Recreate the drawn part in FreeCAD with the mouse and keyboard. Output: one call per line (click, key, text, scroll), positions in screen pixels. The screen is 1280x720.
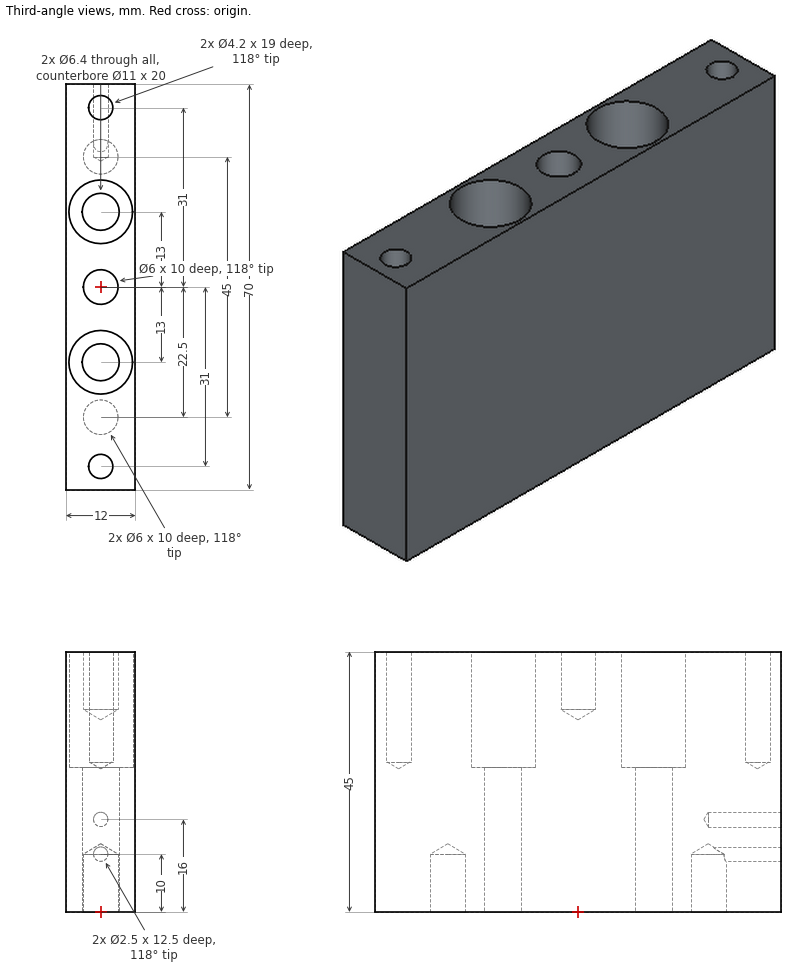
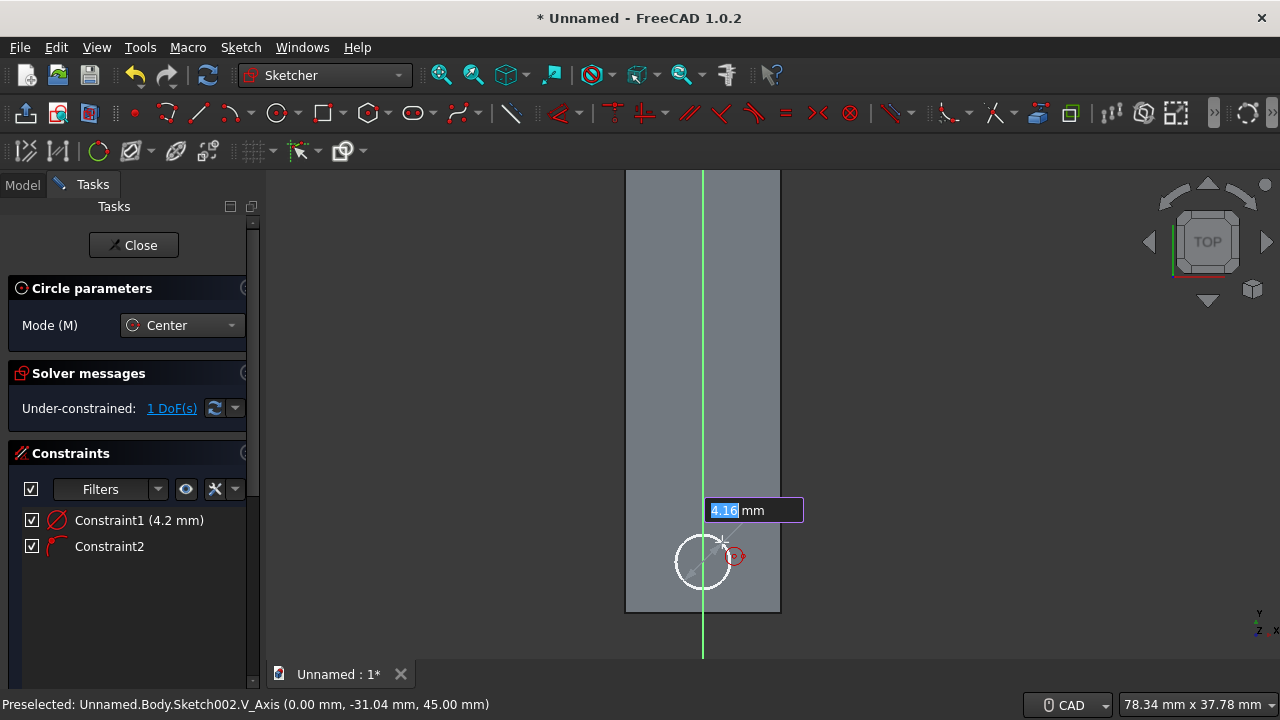
text(4.2)
key(Return)
key(Escape)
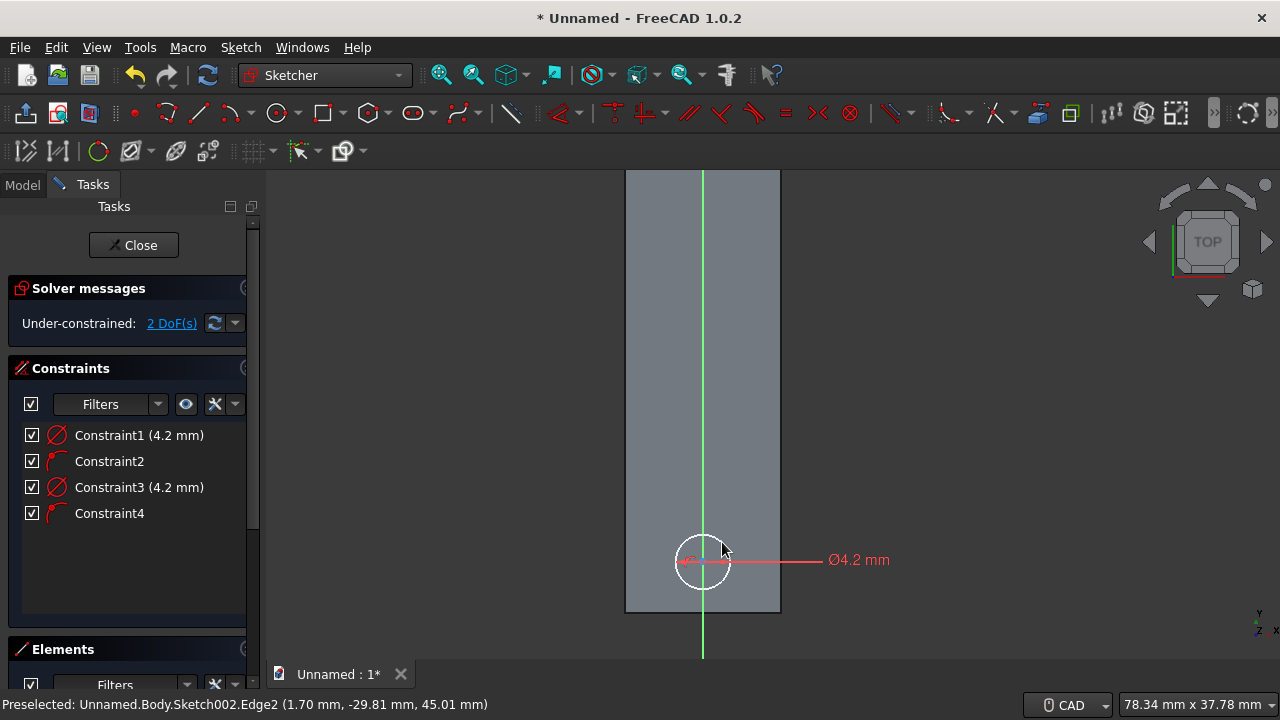
click(558, 114)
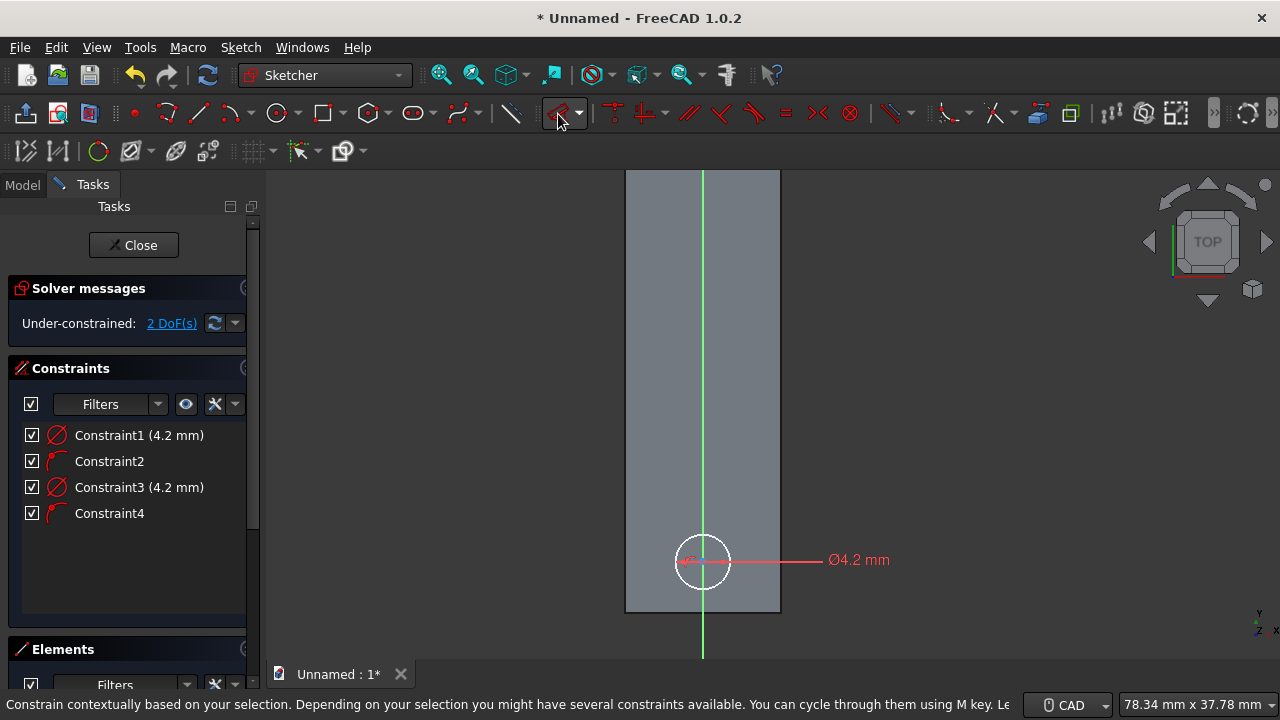
scroll(705, 563, down, 5)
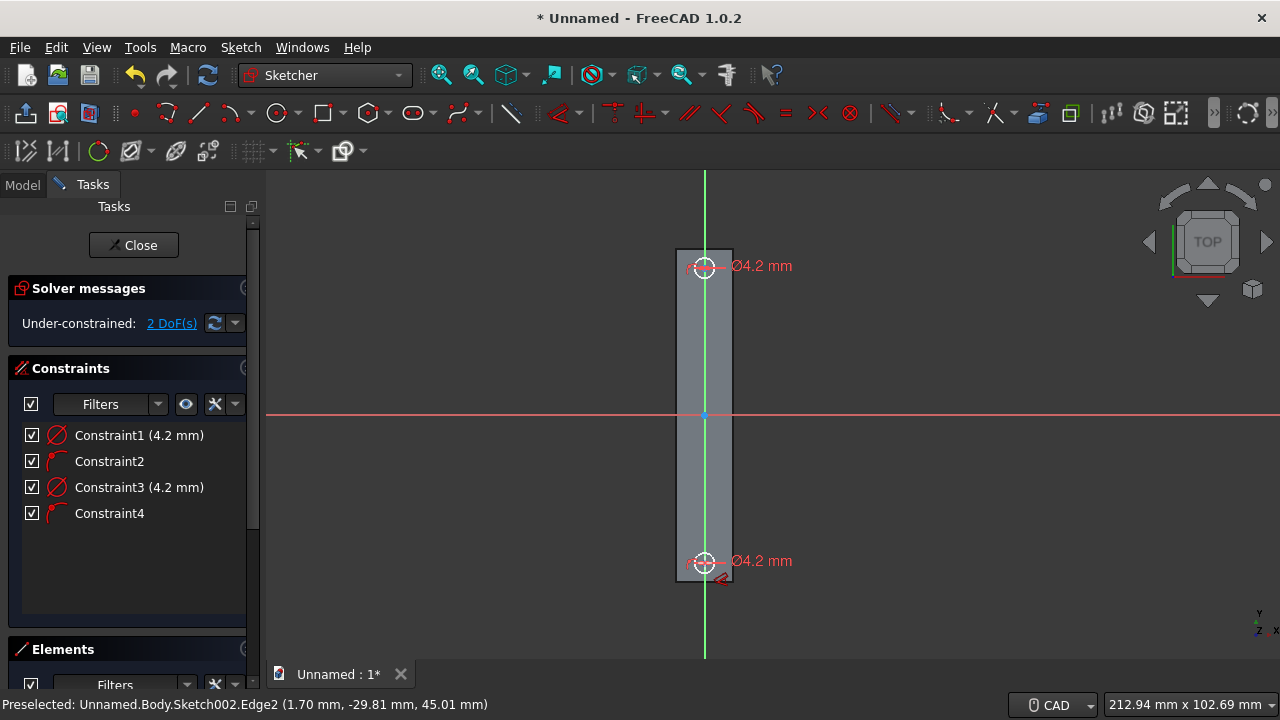
click(705, 268)
click(739, 342)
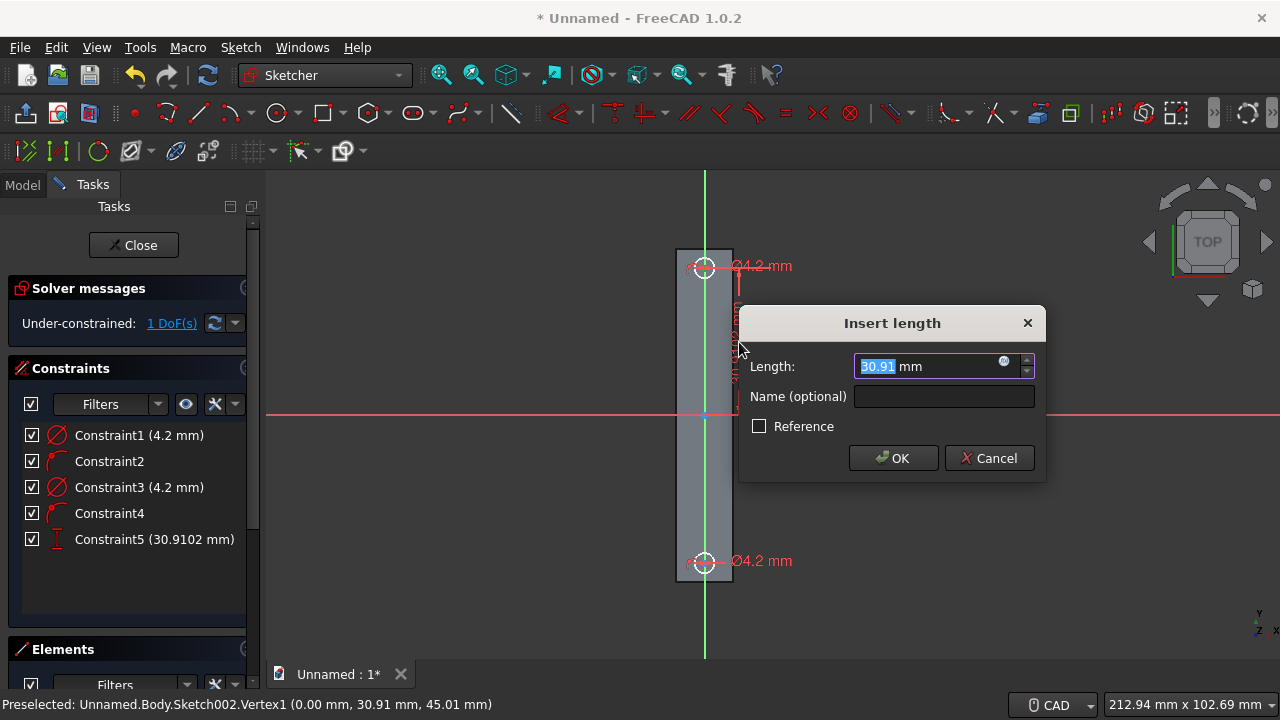
text(31)
key(Return)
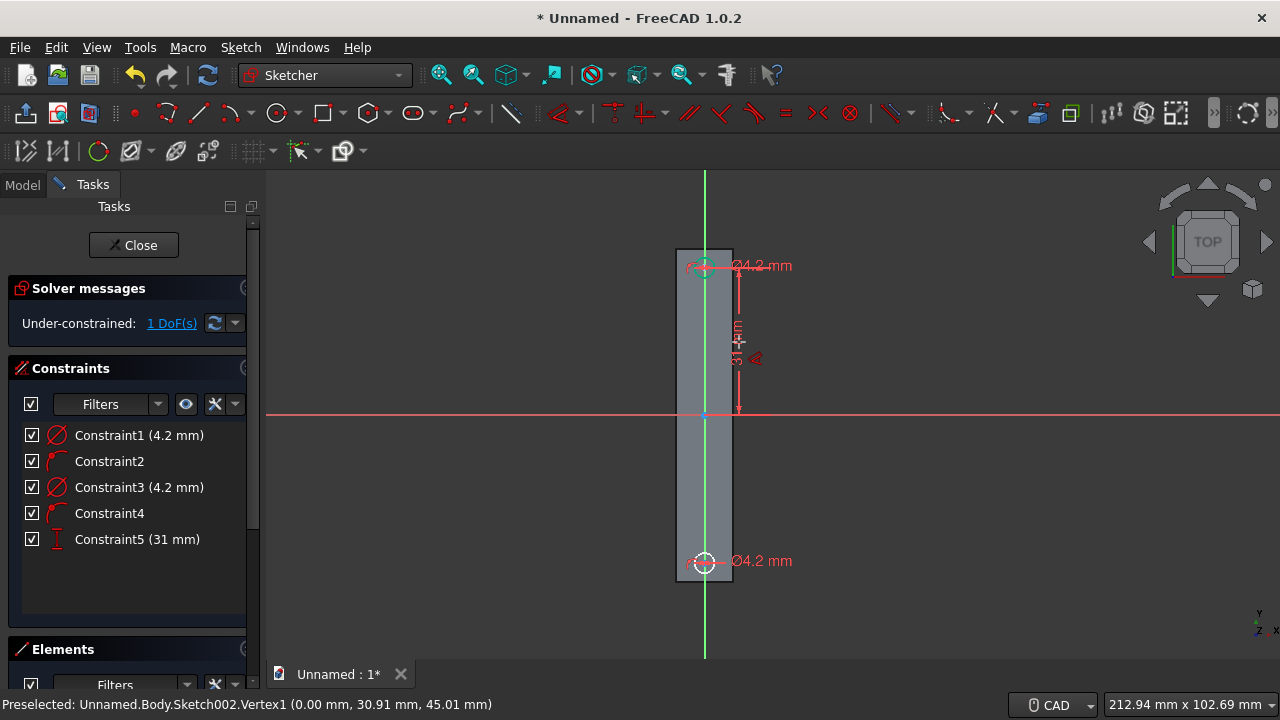
click(705, 563)
click(739, 489)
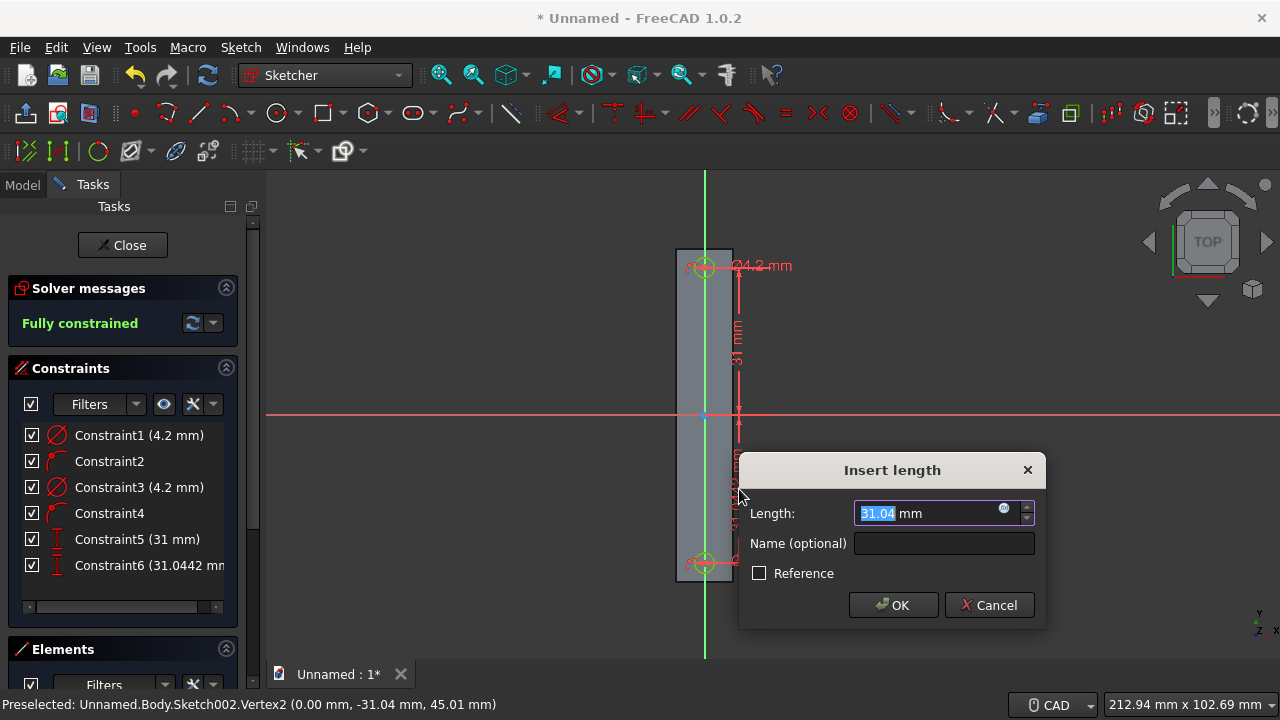
text(31)
key(Return)
key(Escape)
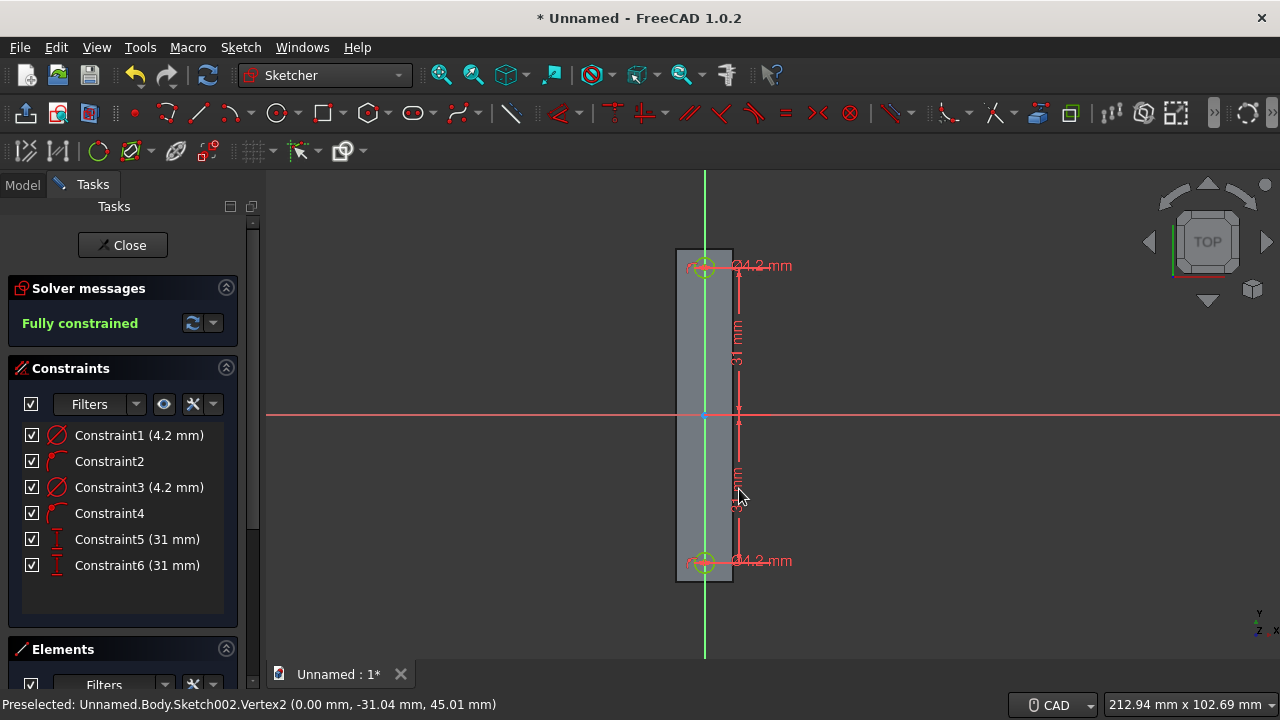
click(123, 245)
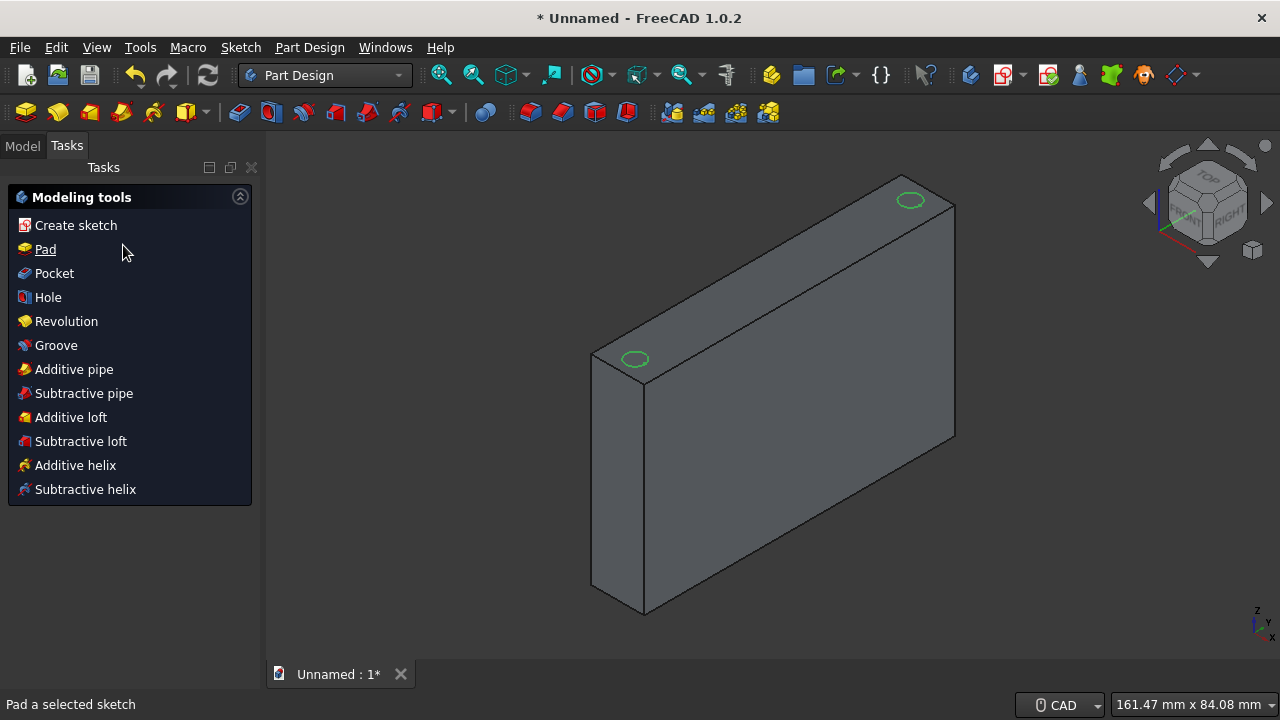
click(272, 112)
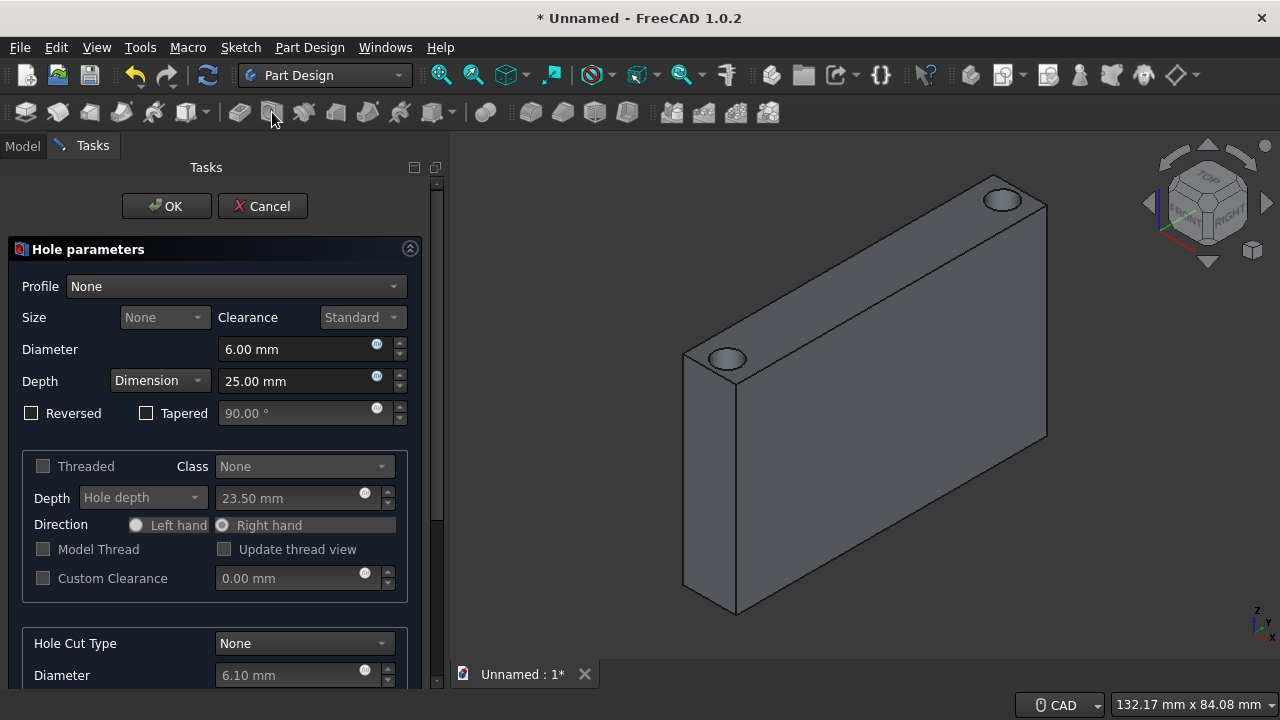
triple_click(305, 349)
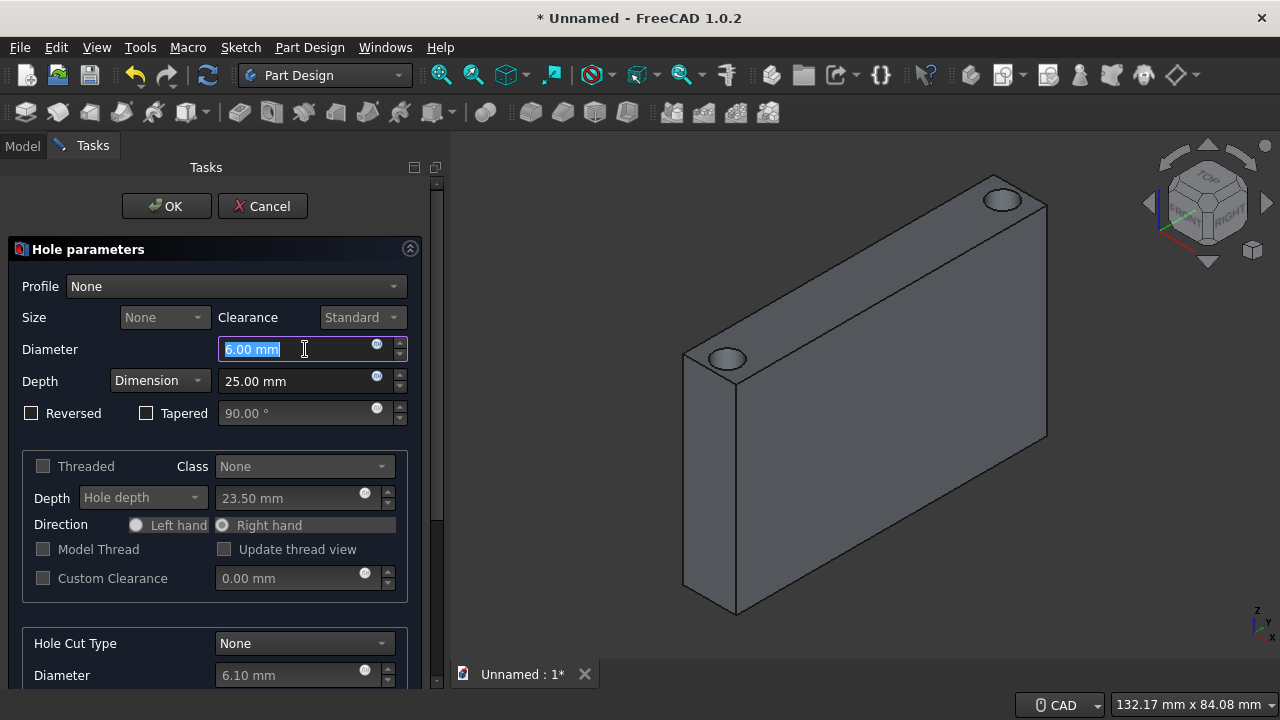
text(4.2)
key(Tab)